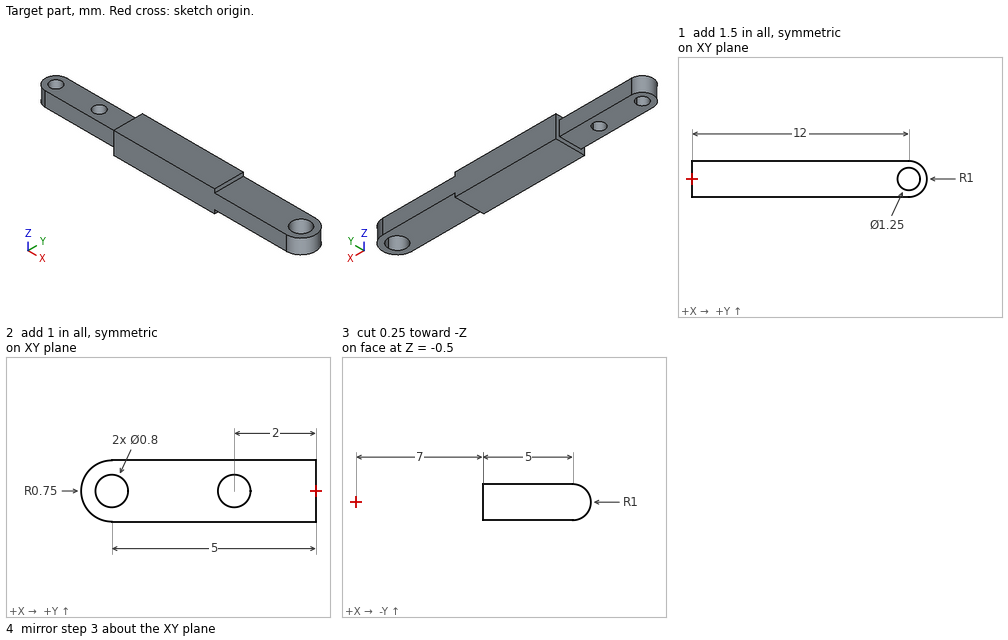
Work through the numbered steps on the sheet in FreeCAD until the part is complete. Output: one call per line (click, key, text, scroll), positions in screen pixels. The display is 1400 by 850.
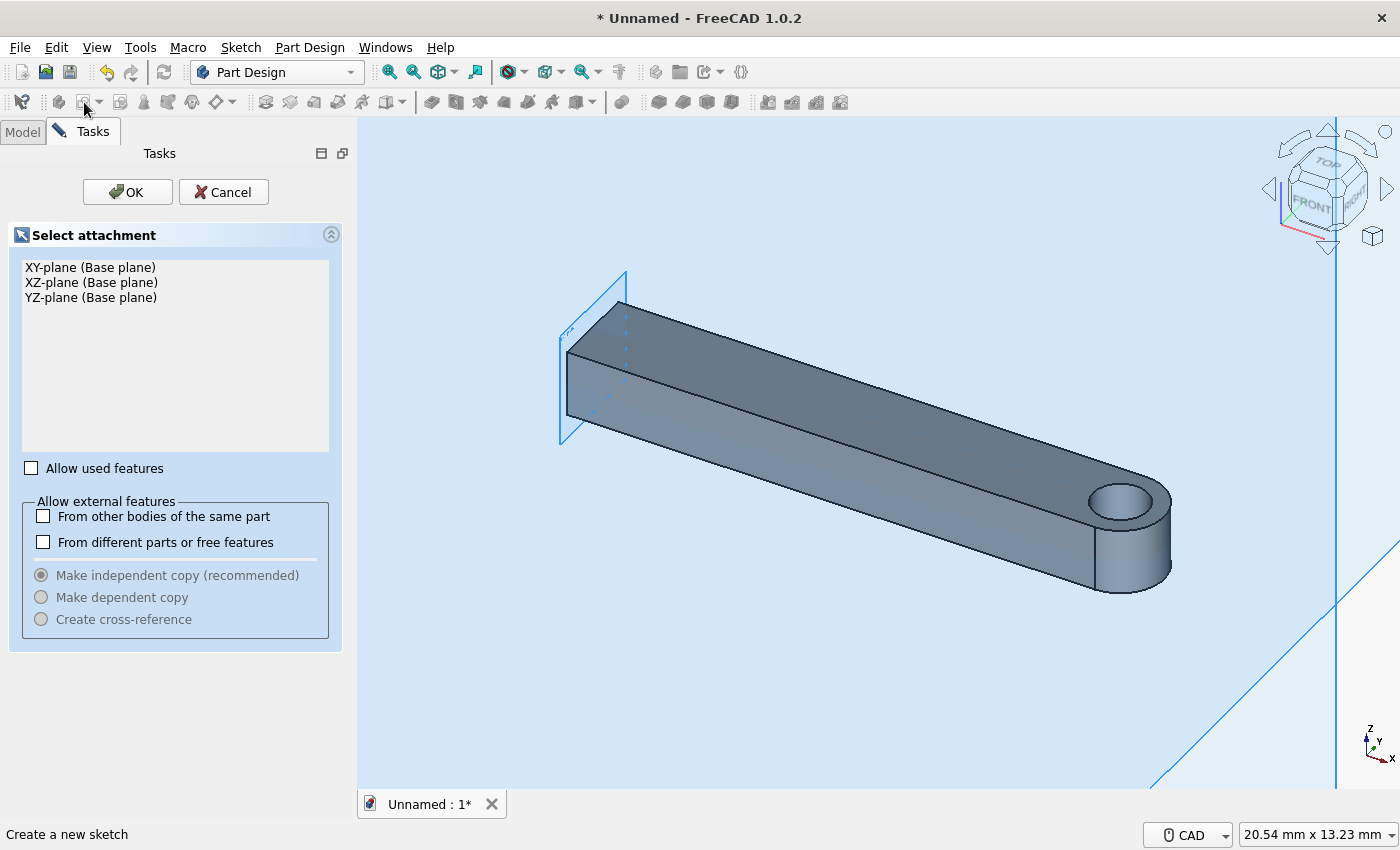
click(82, 268)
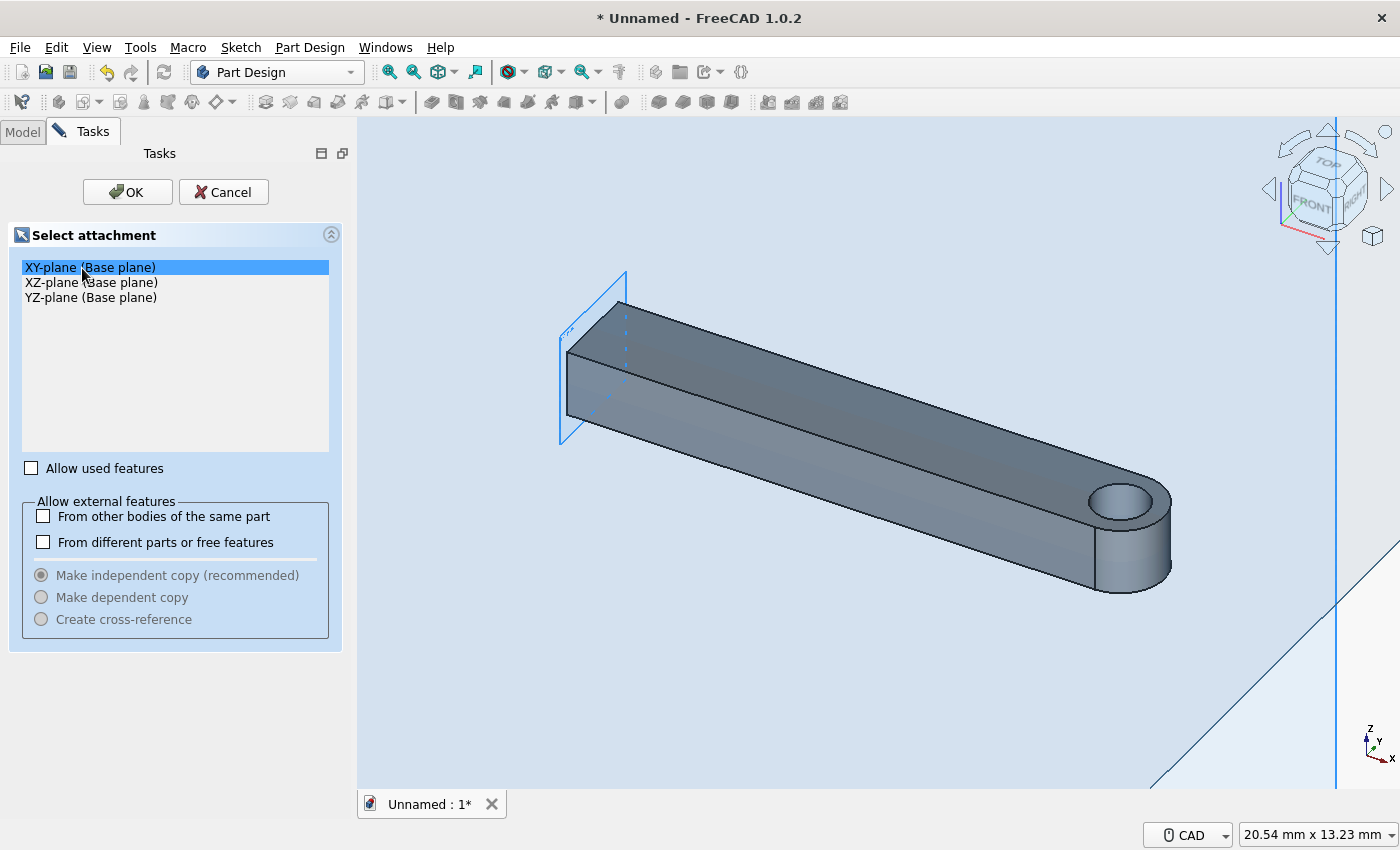
click(128, 192)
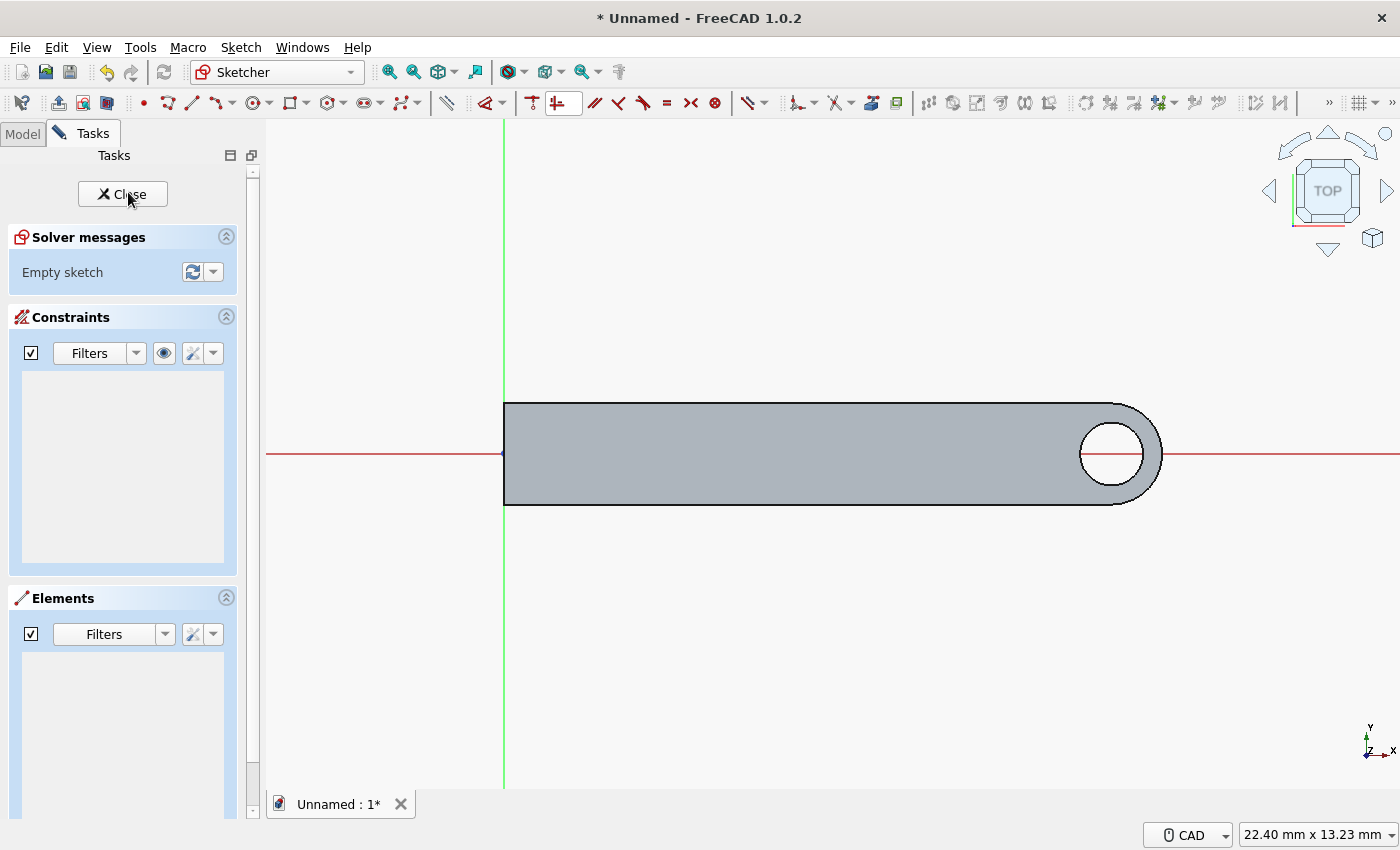
click(108, 104)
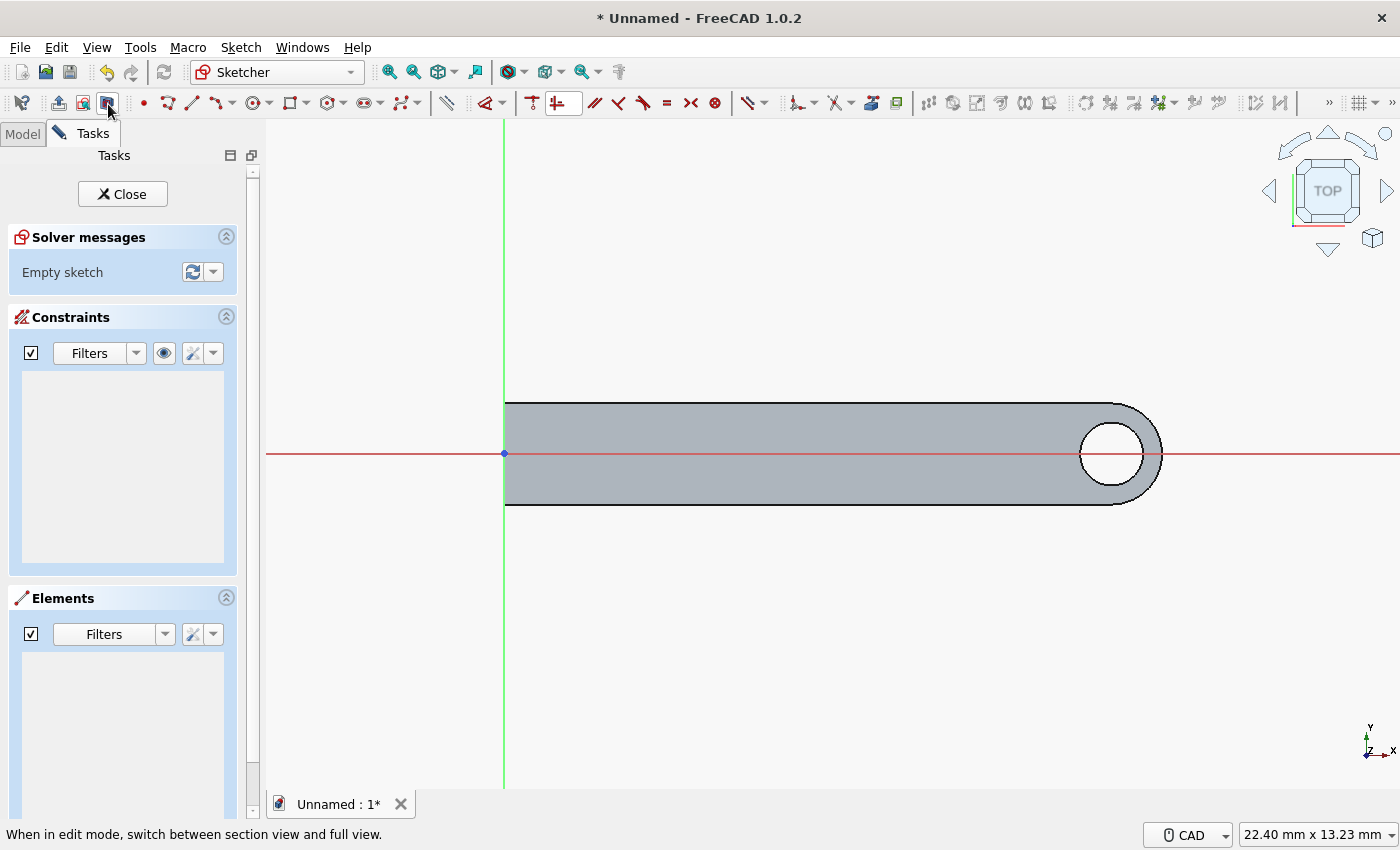
scroll(764, 454, down, 5)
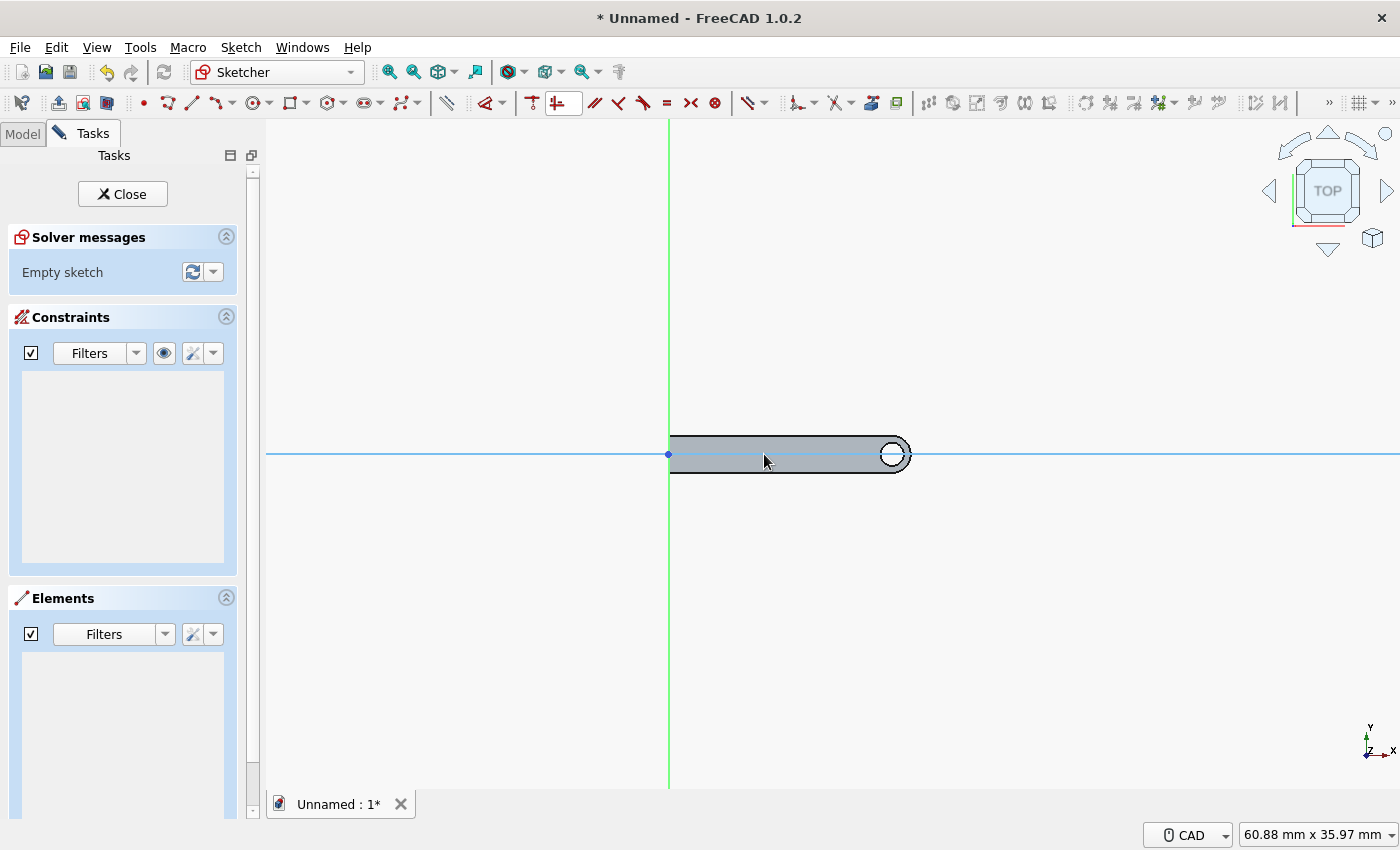
scroll(586, 454, up, 9)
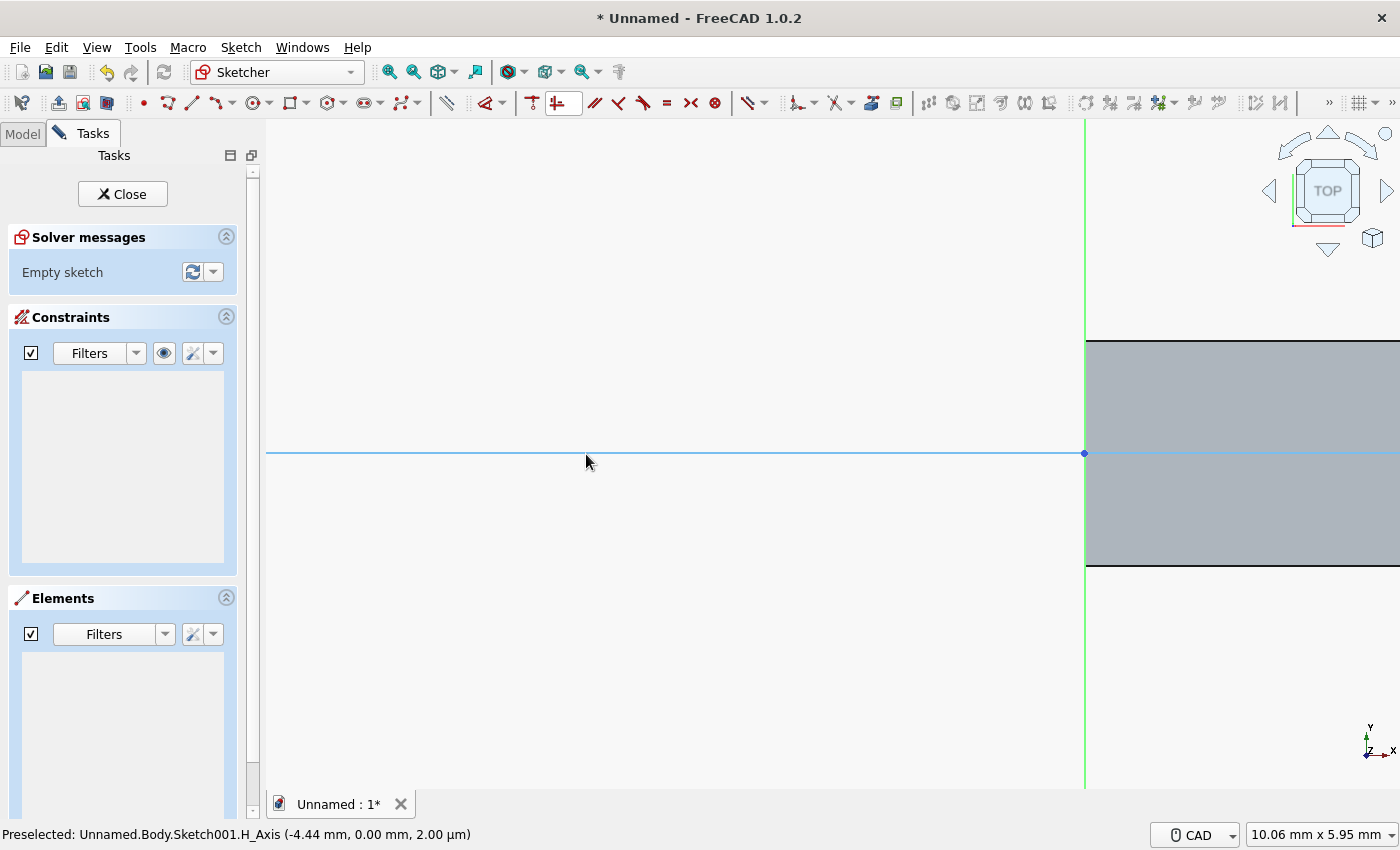
click(168, 104)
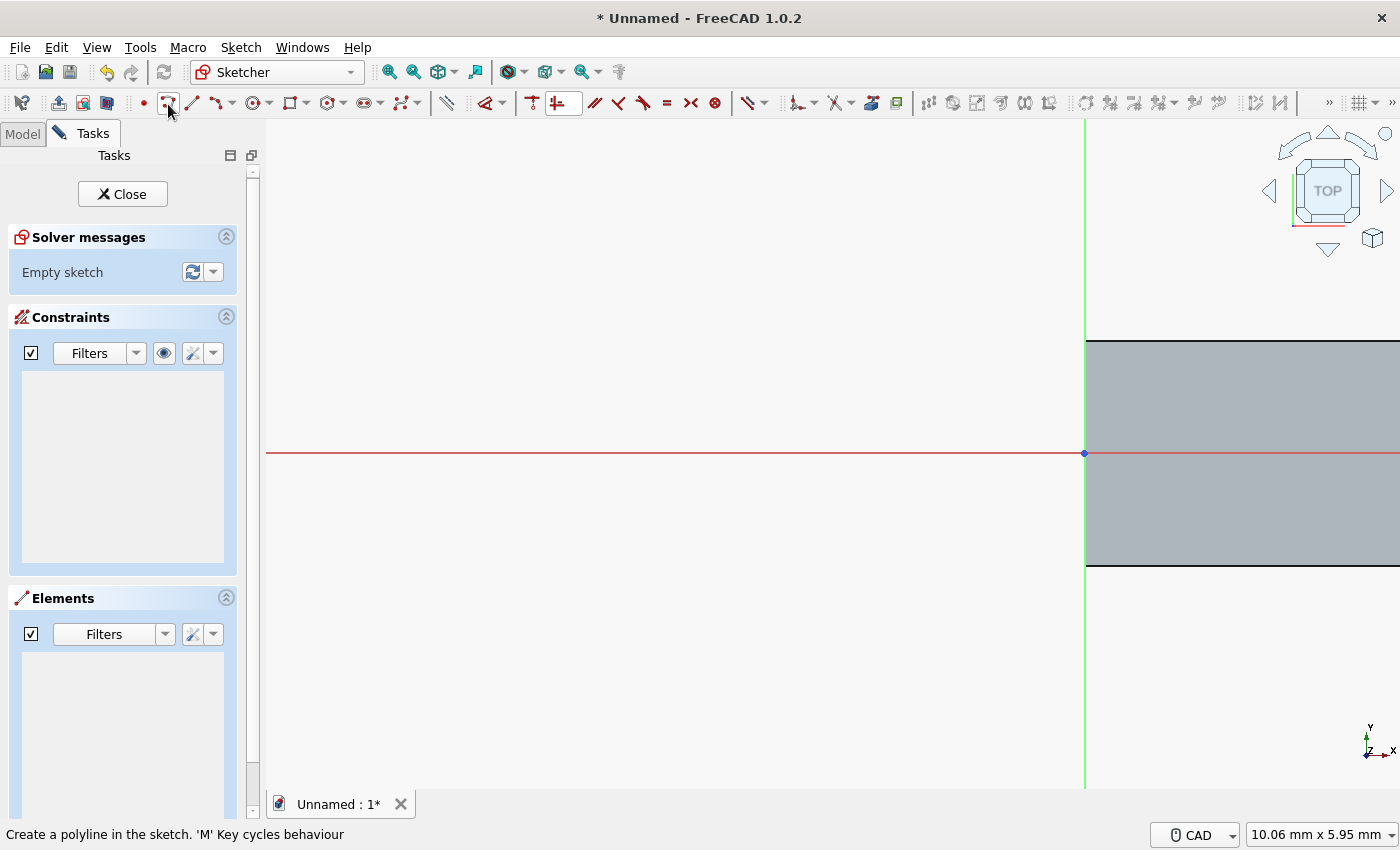
click(521, 538)
click(1085, 538)
click(1076, 369)
click(521, 369)
right_click(521, 369)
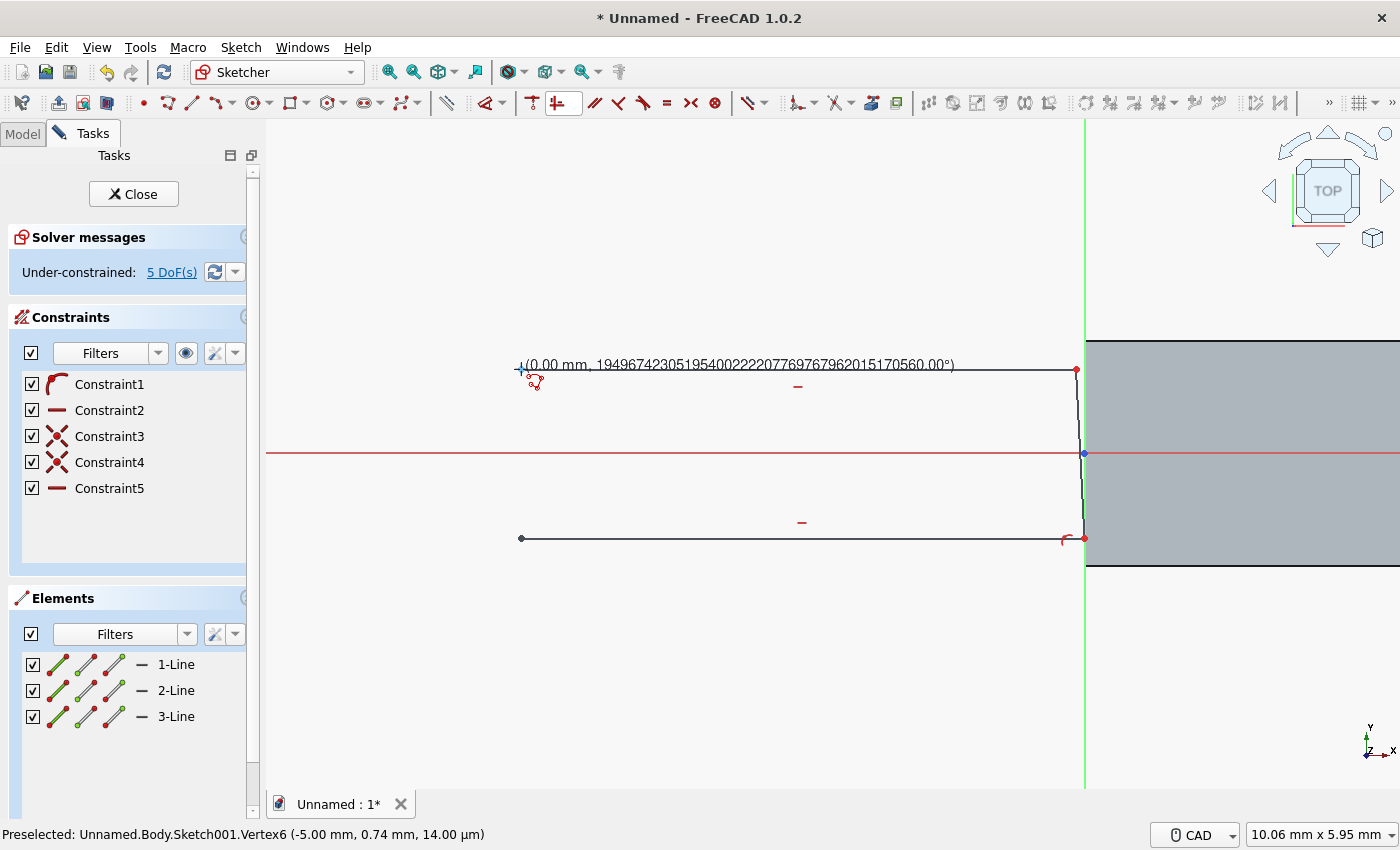
click(216, 104)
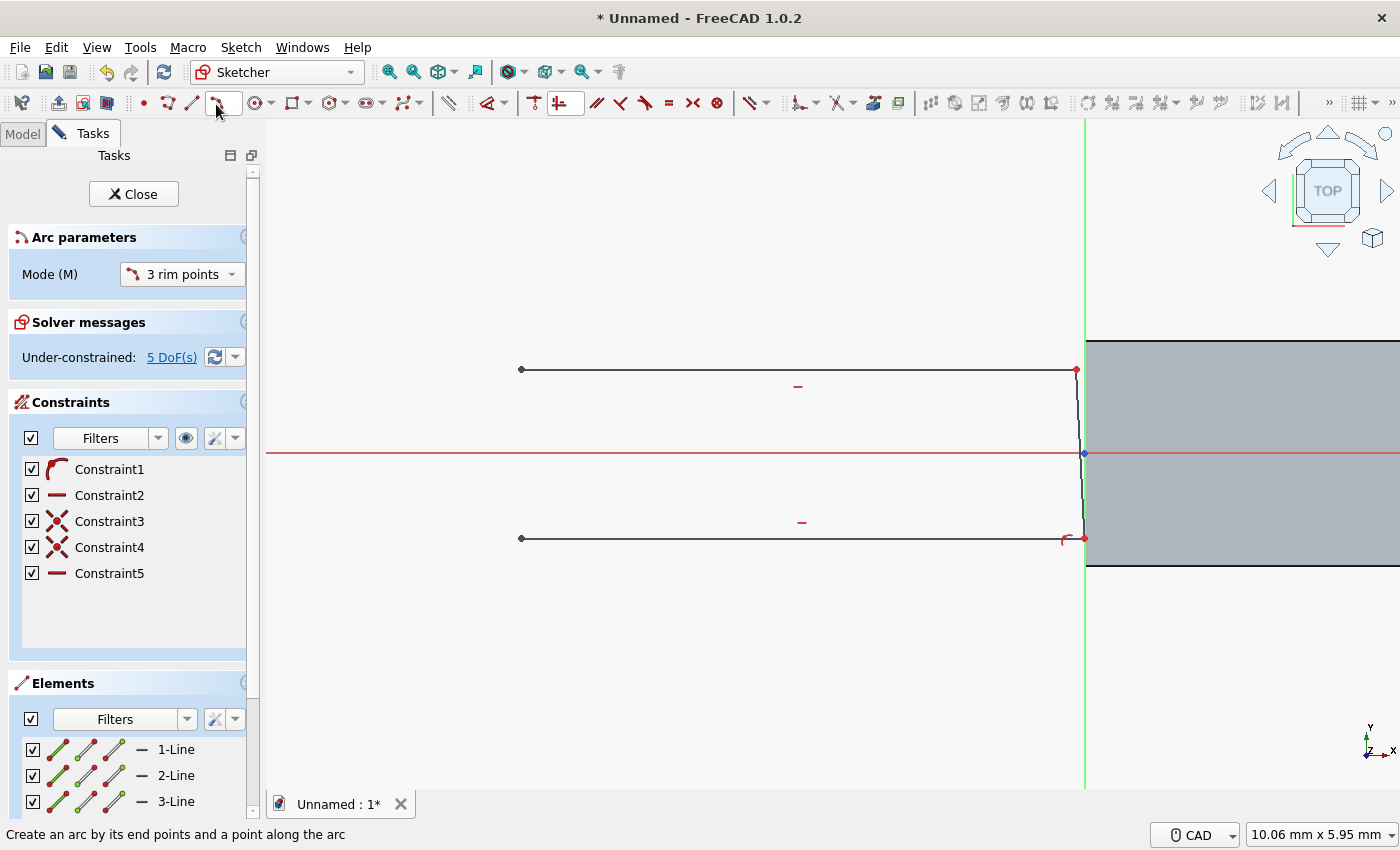
click(521, 370)
click(521, 539)
click(441, 427)